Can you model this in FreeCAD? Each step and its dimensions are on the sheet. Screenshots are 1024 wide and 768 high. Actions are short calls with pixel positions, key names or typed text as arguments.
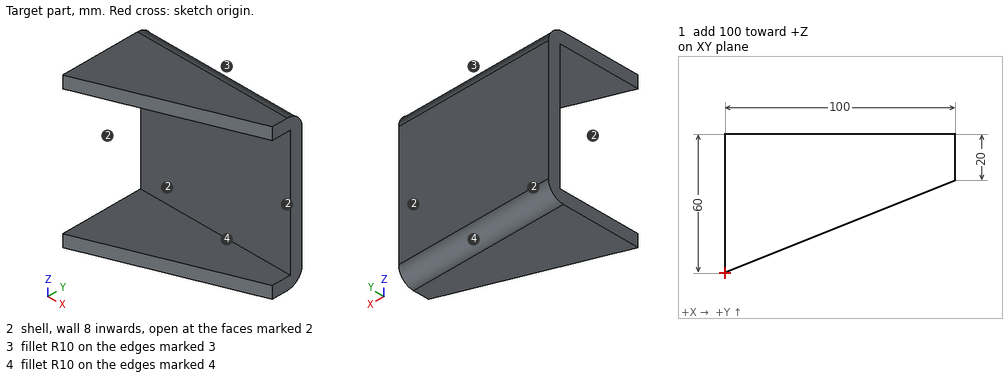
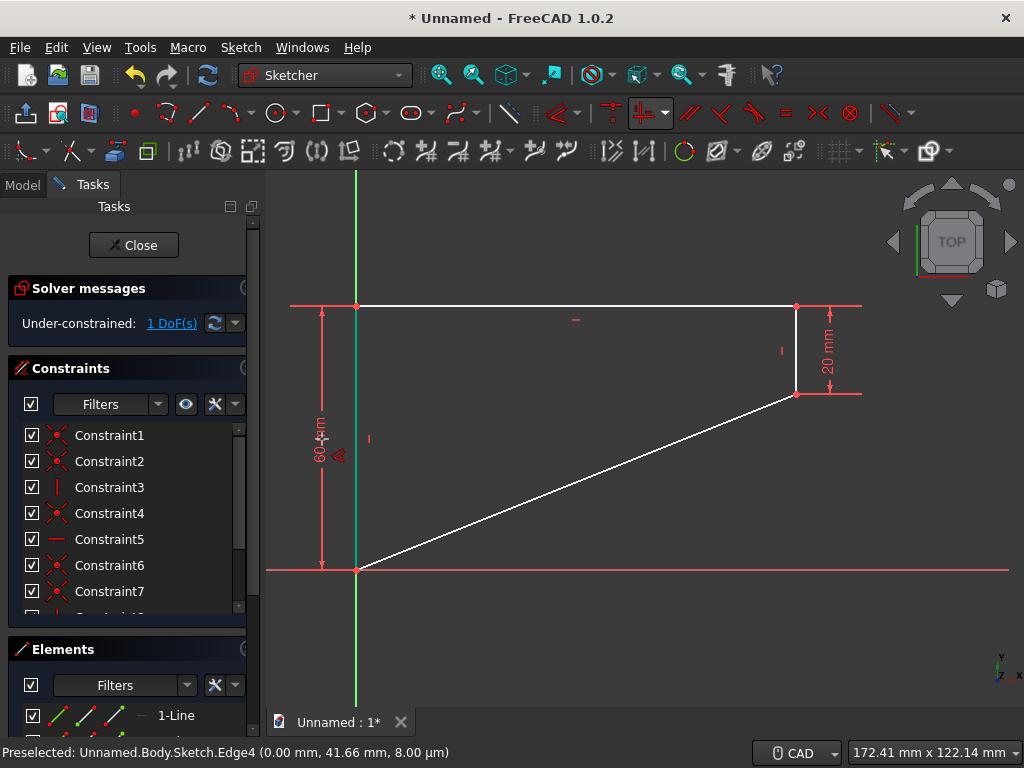
click(664, 306)
click(576, 272)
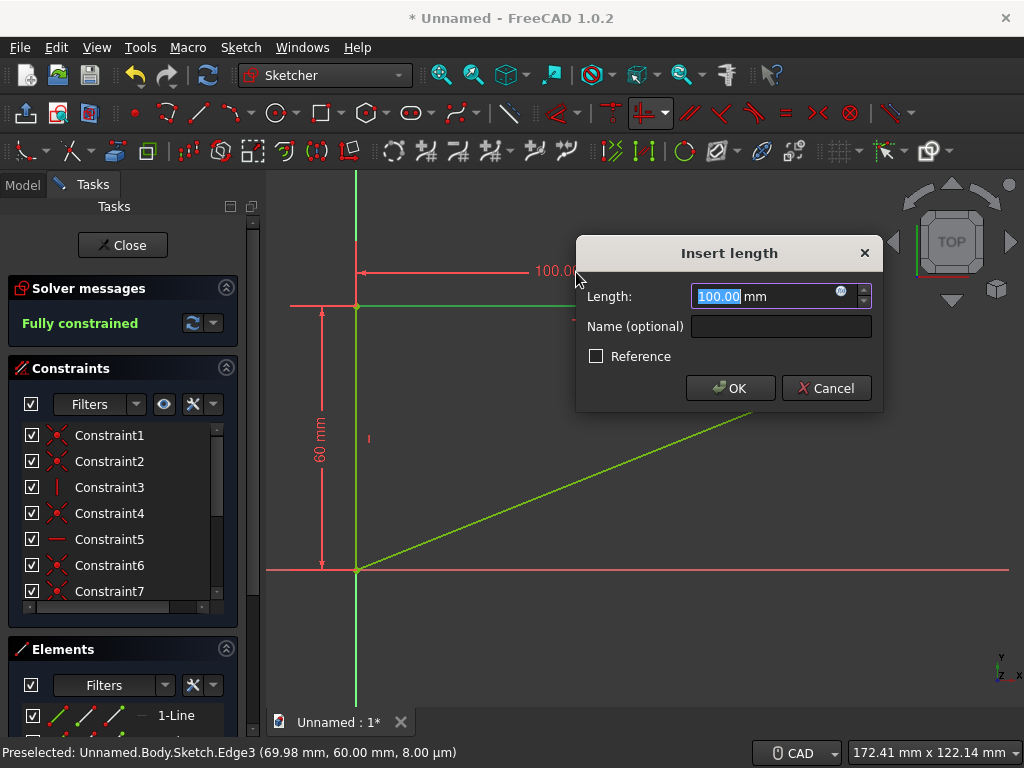
text(100)
key(Return)
key(Escape)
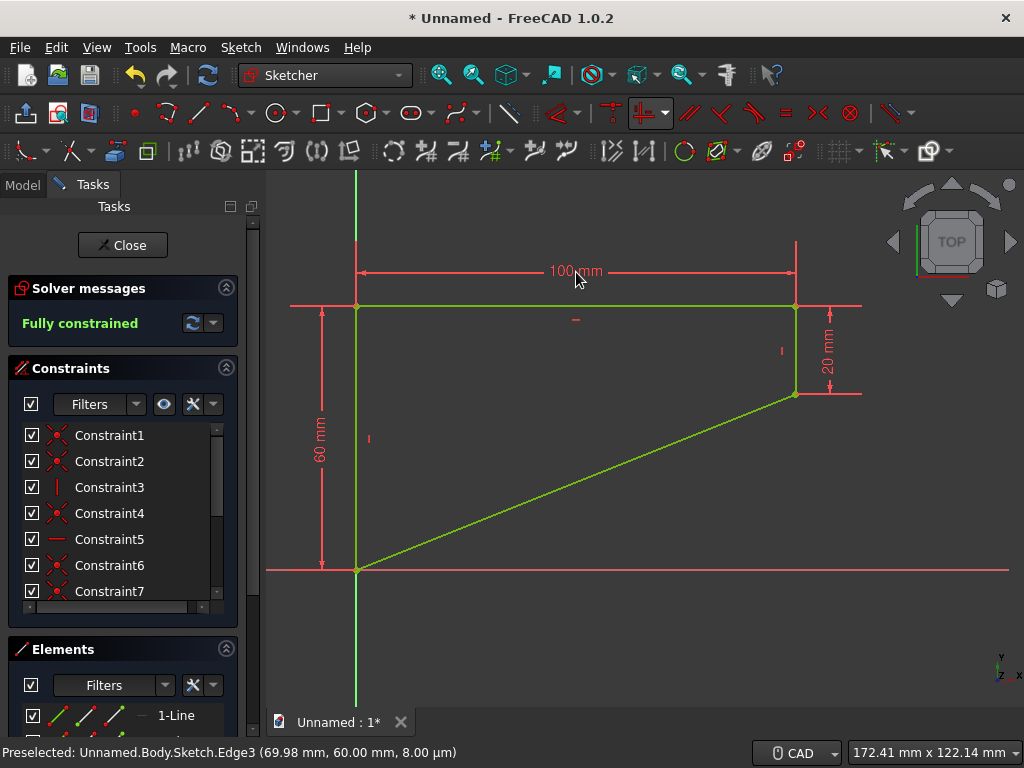
click(123, 245)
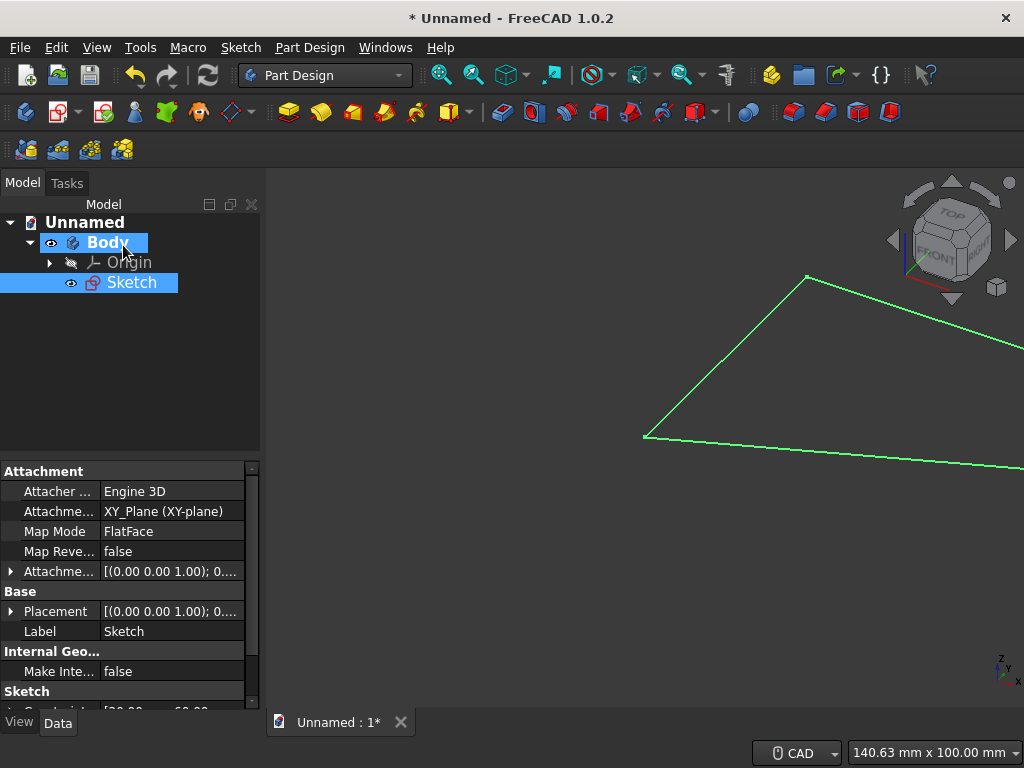
click(290, 112)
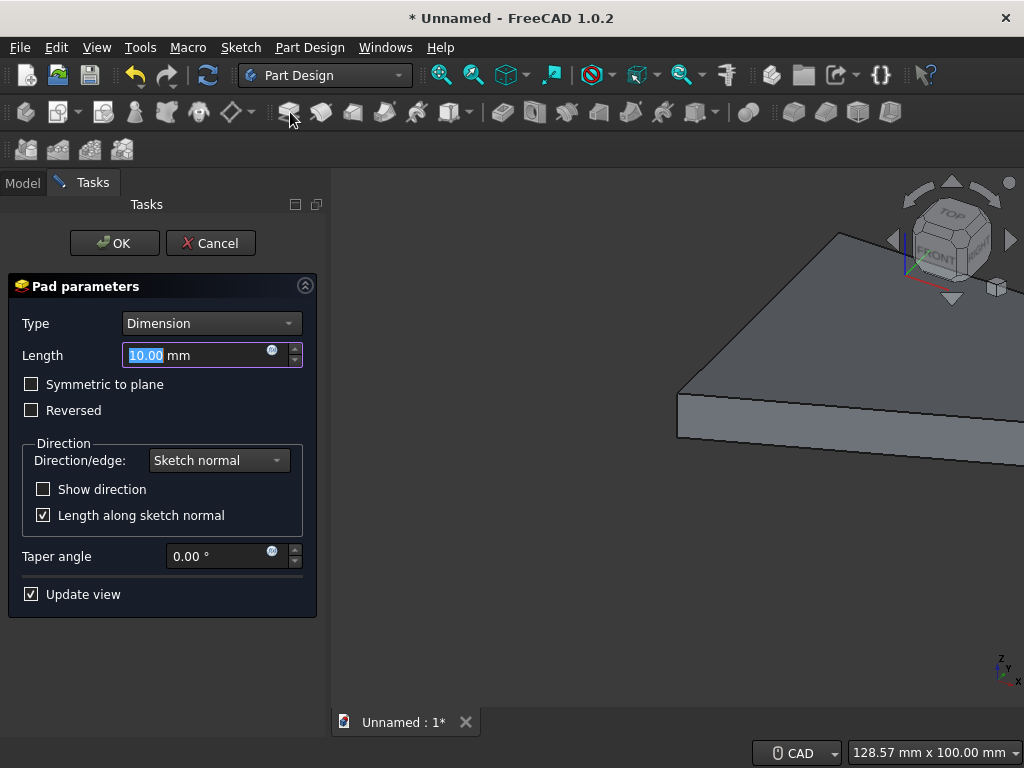
text(100)
key(Tab)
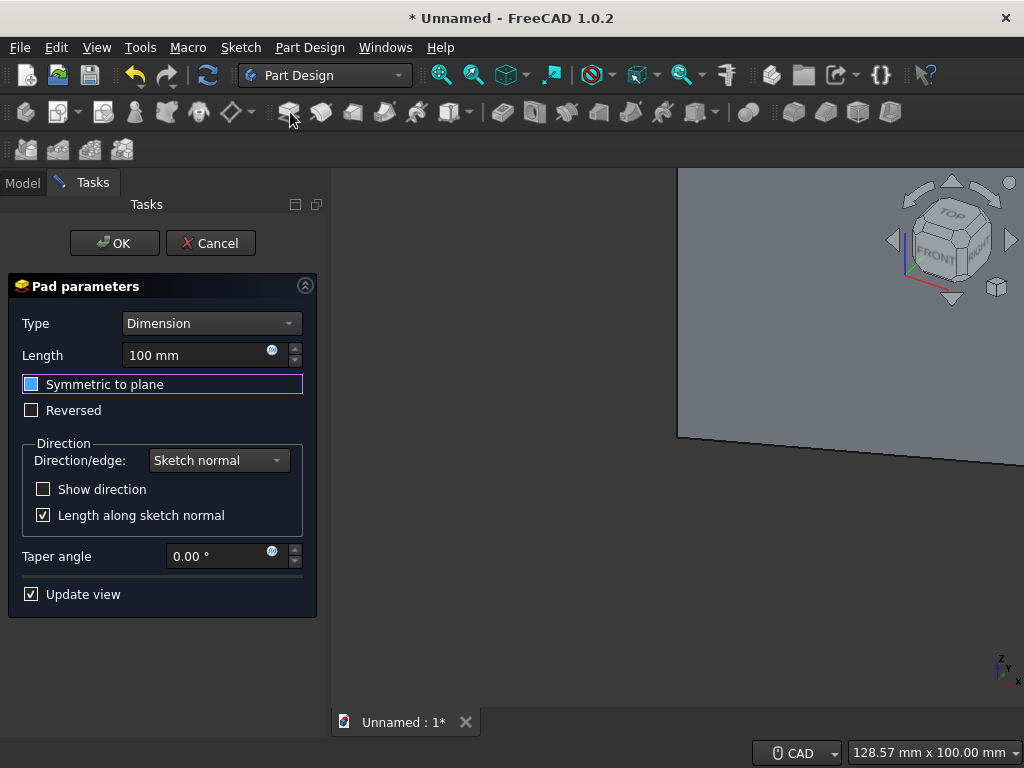
click(115, 243)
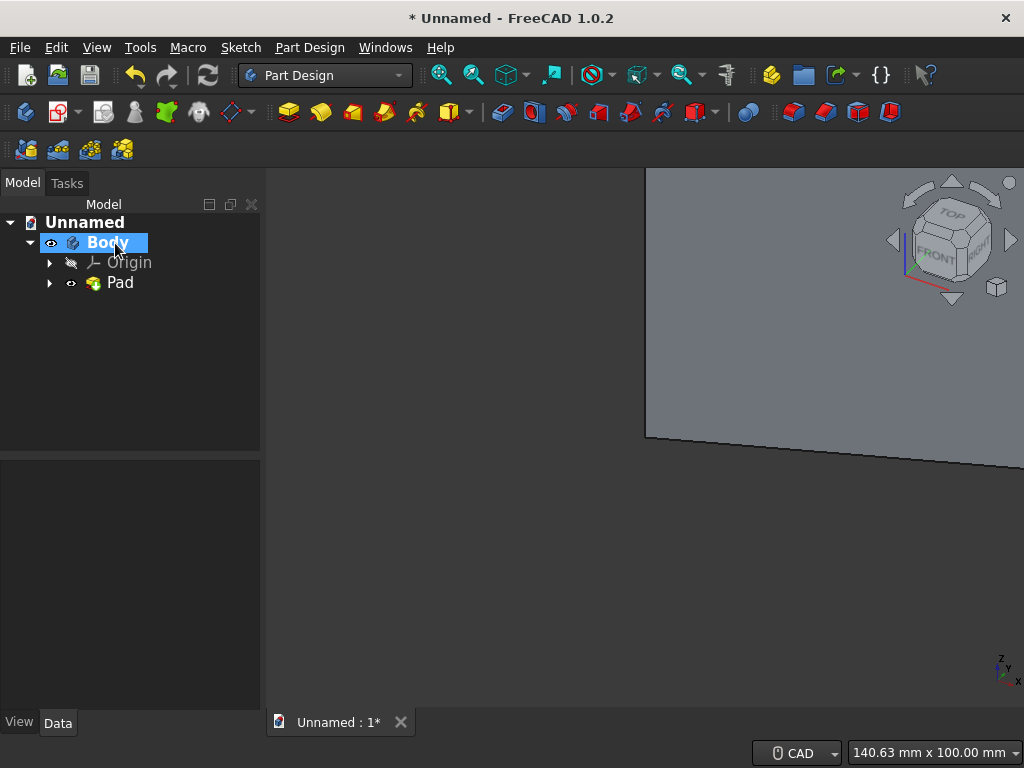
click(442, 76)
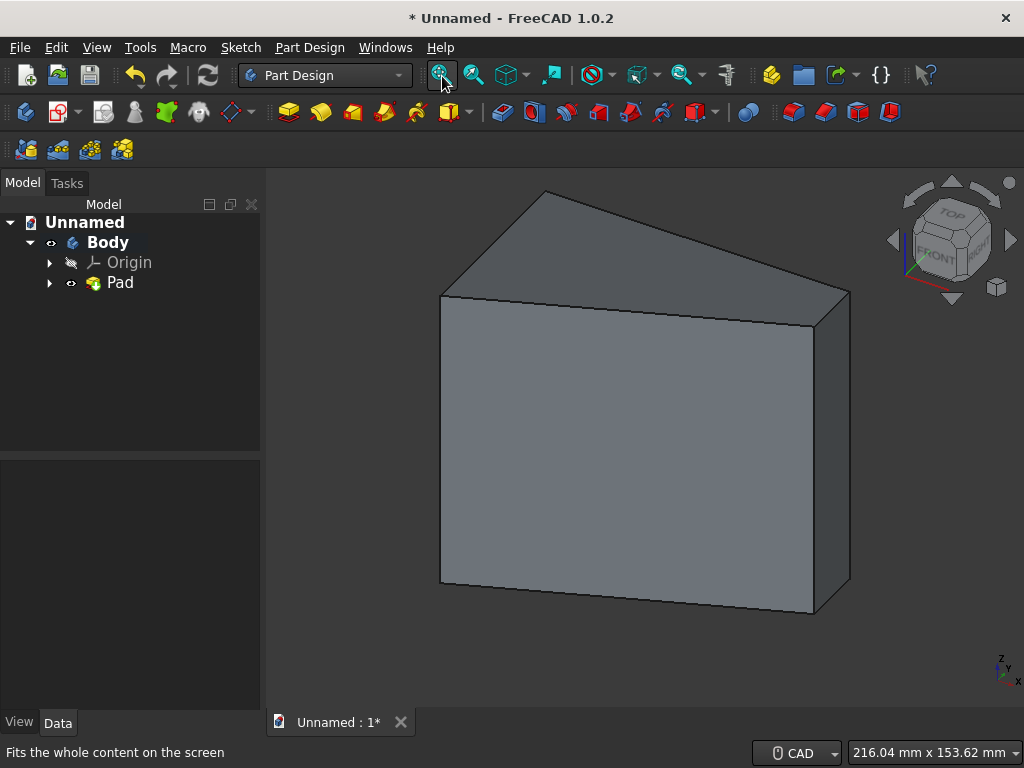
click(832, 370)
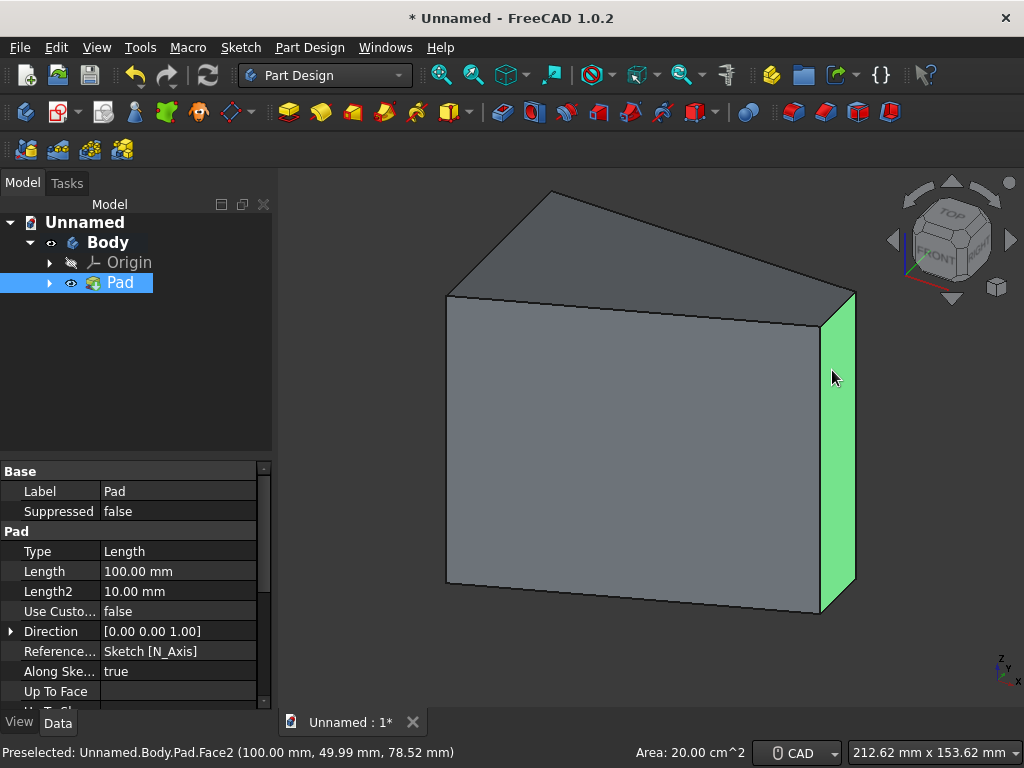
click(633, 454, ctrl)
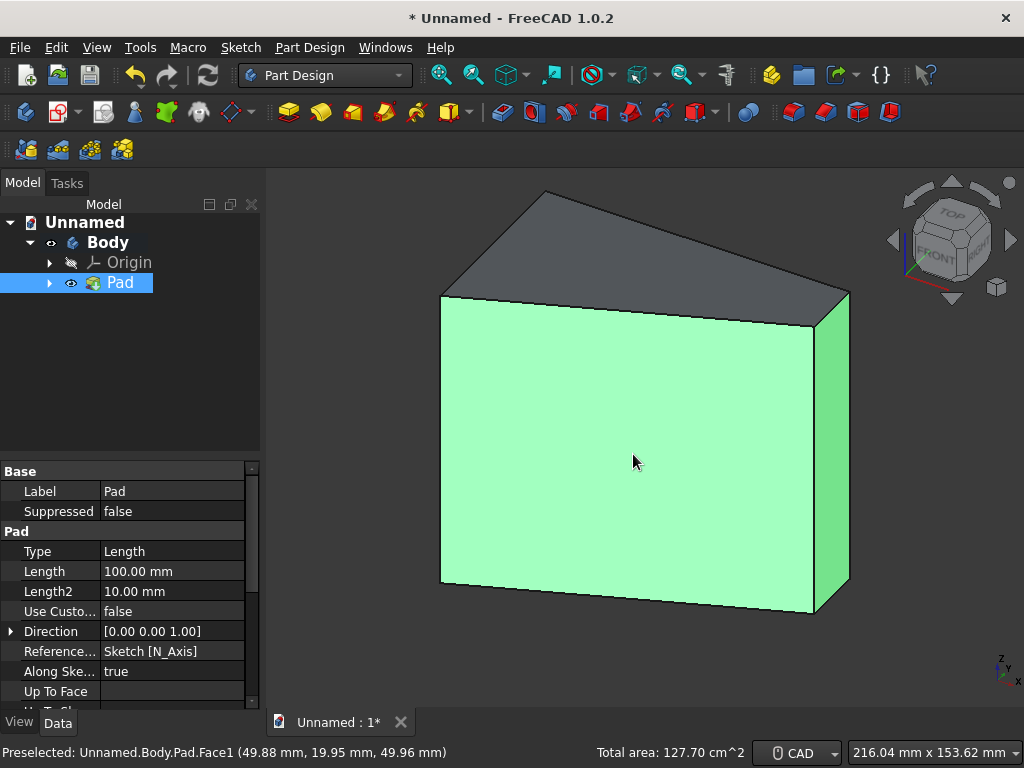
key(0)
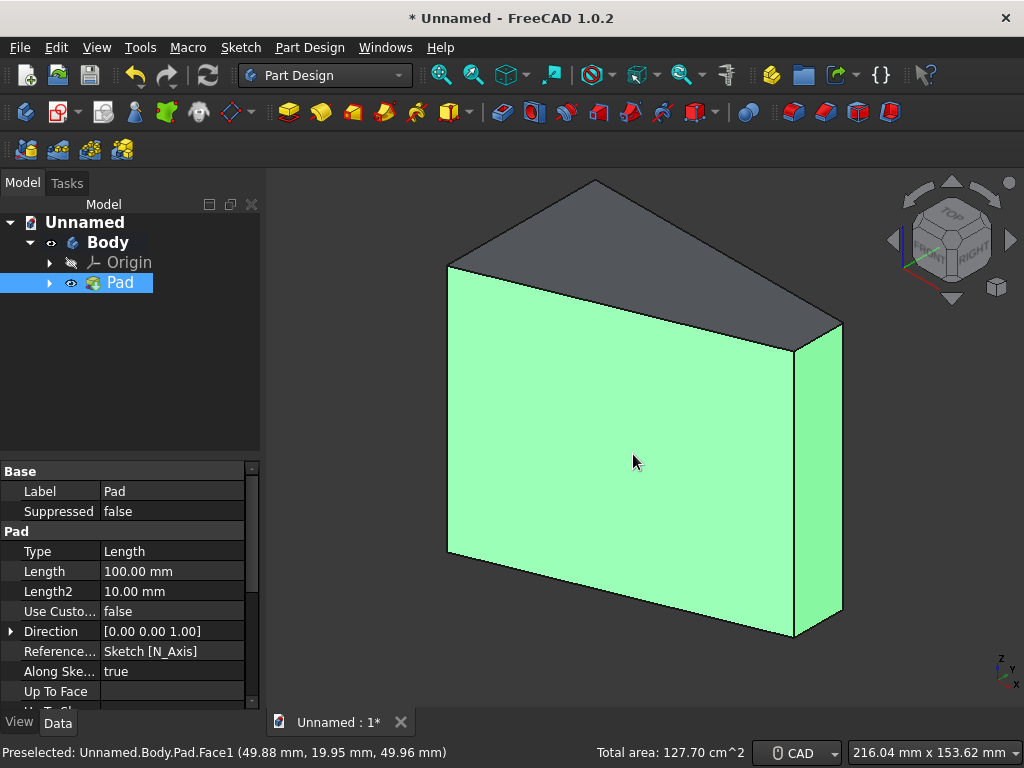
key(2)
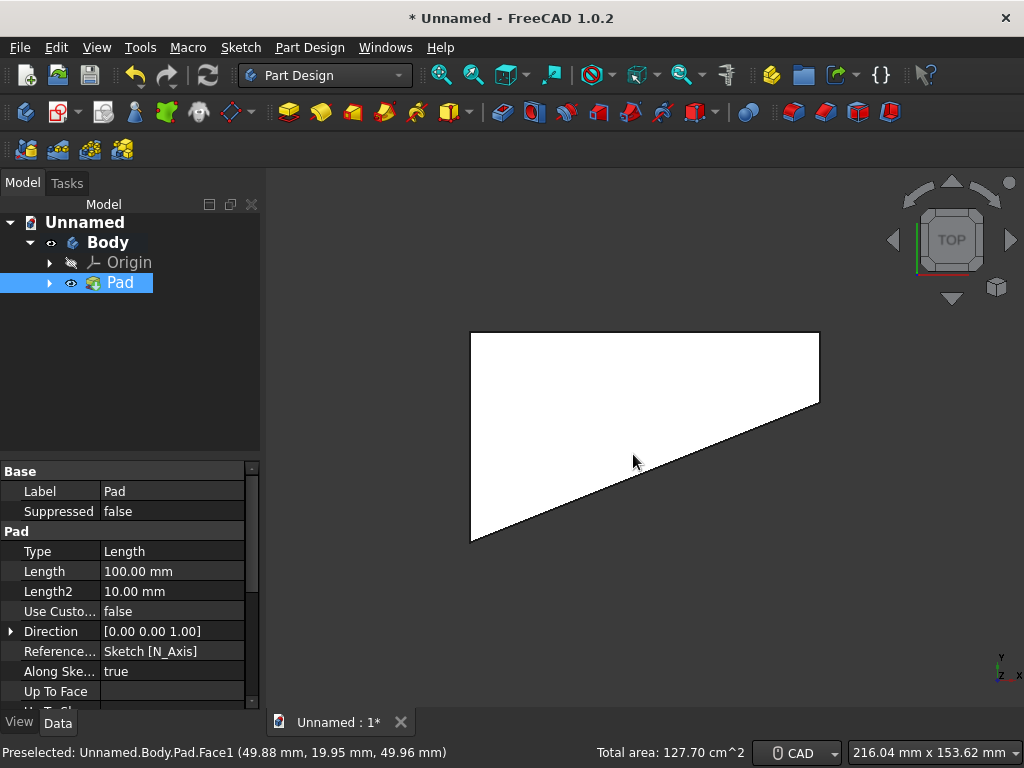
key(1)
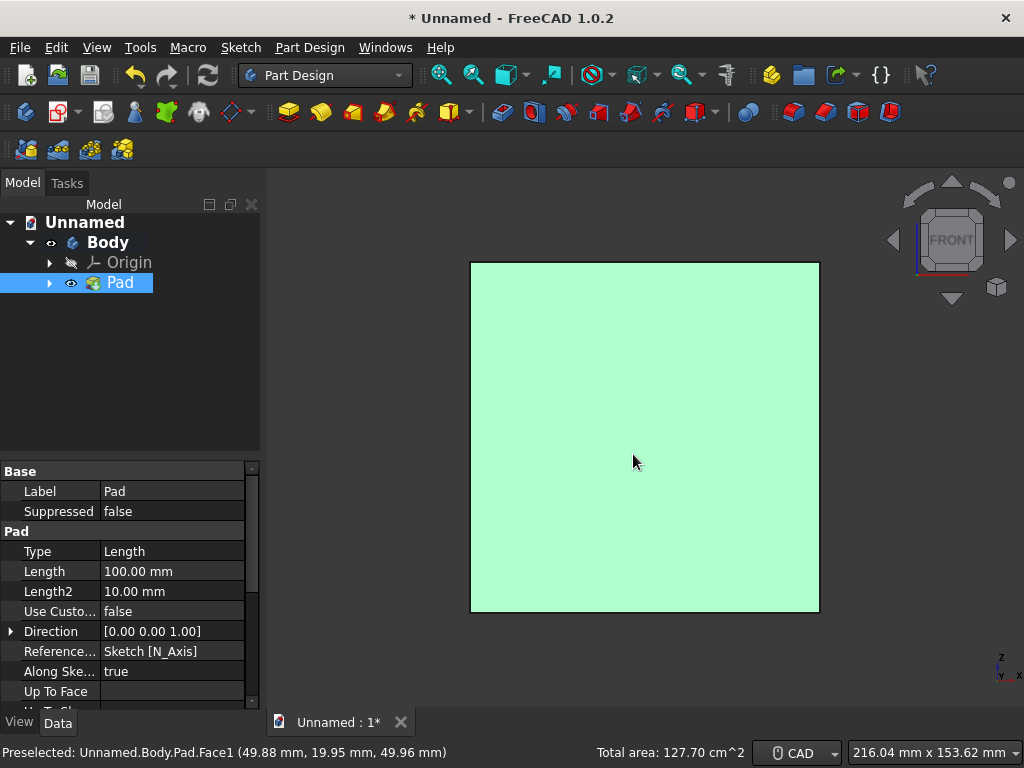
key(3)